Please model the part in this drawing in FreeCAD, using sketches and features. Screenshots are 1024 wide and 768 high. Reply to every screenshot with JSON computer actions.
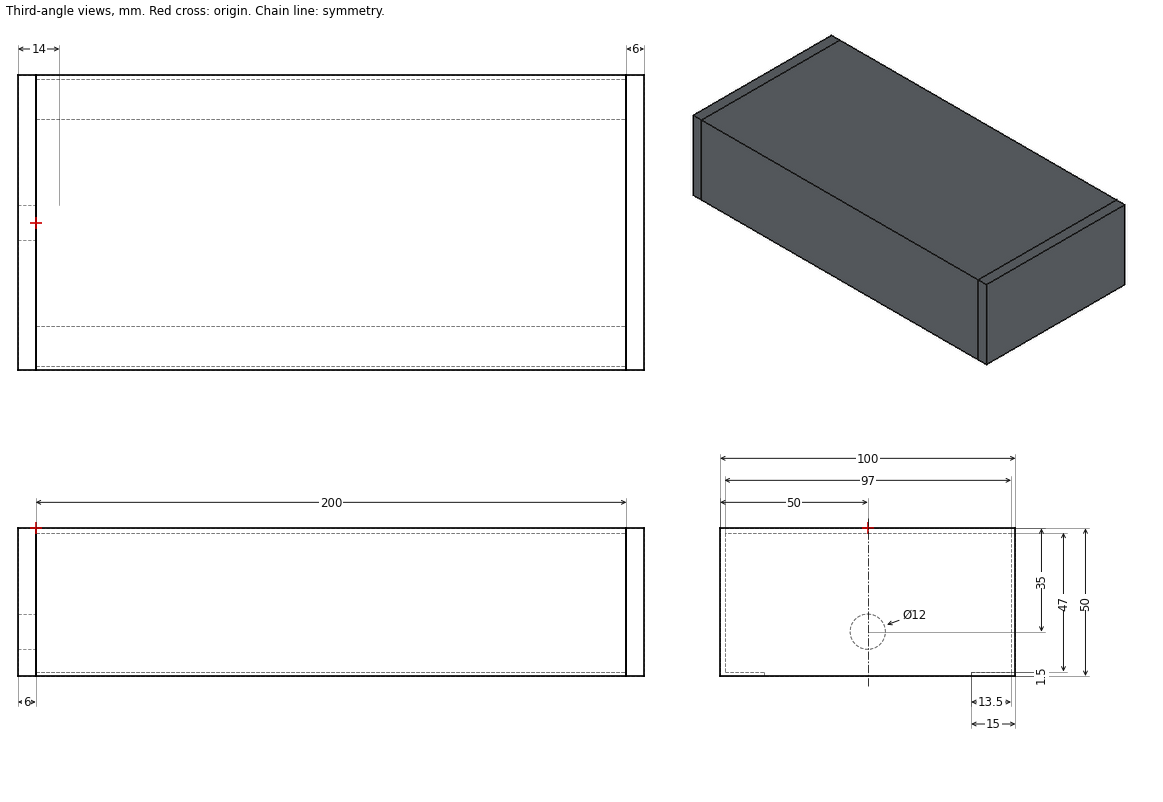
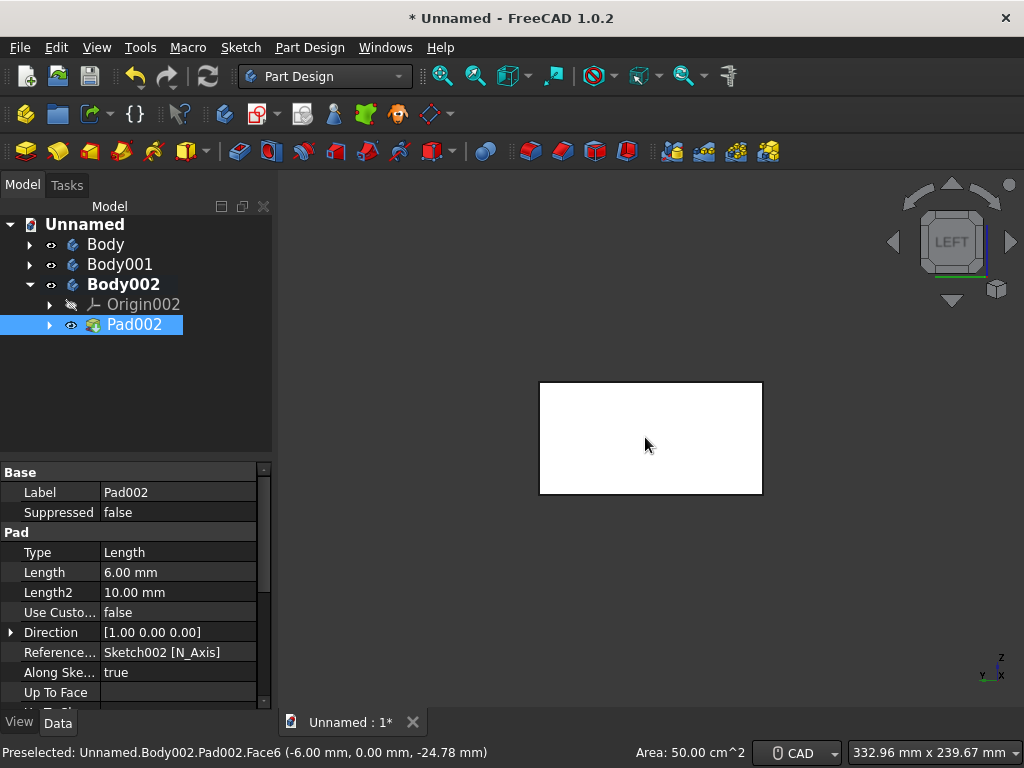
{"action": "left_click", "coordinate": [258, 114]}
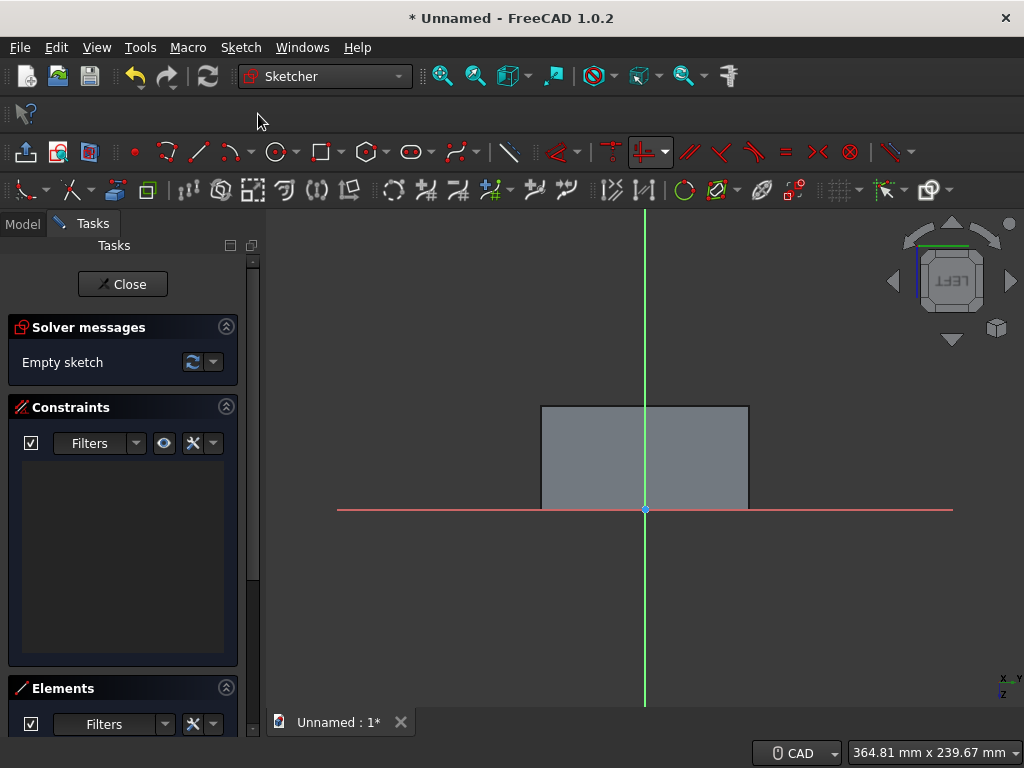
{"action": "scroll", "coordinate": [650, 436], "scroll_direction": "up", "scroll_amount": 13}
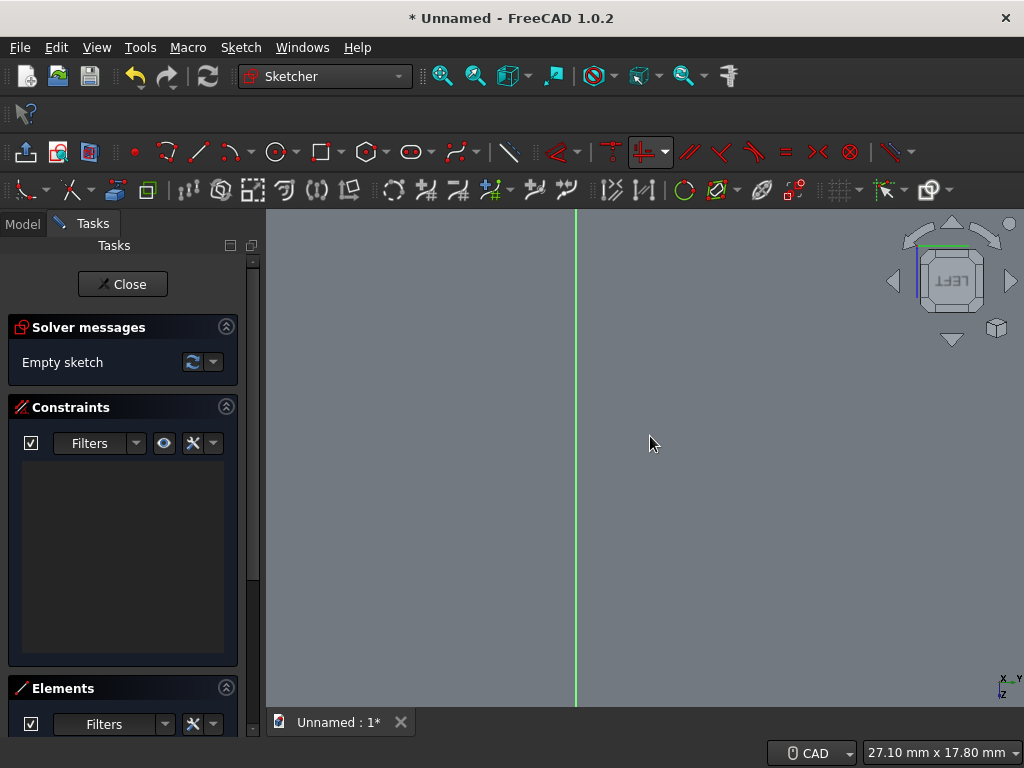
{"action": "left_click", "coordinate": [276, 152]}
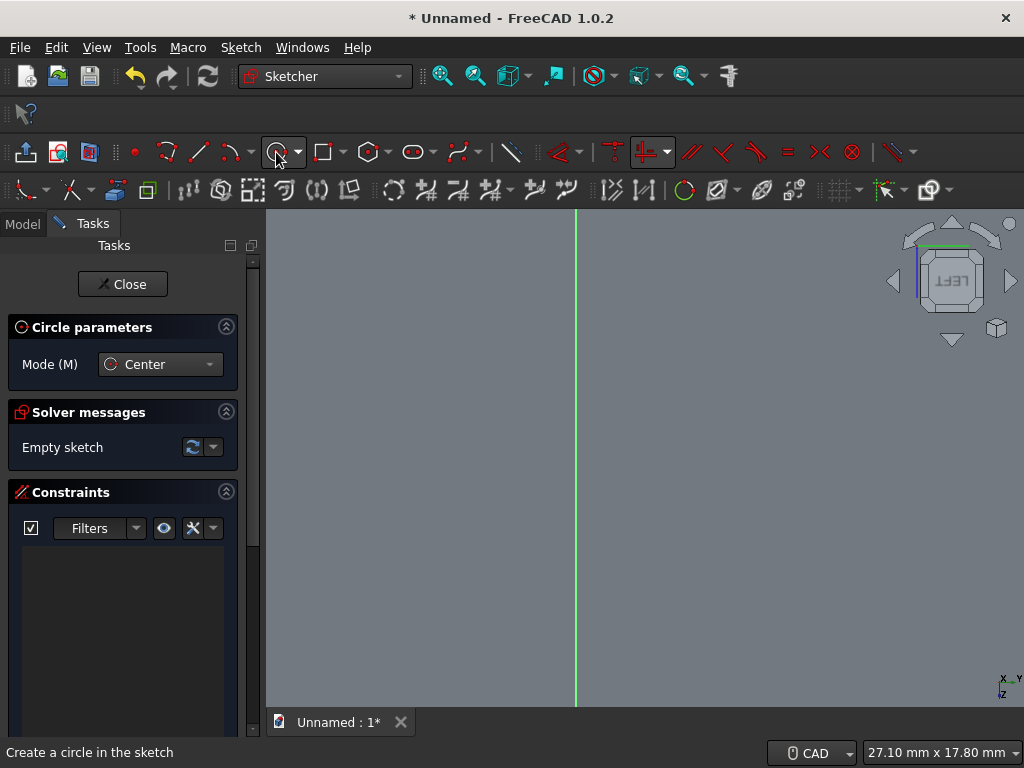
{"action": "left_click", "coordinate": [576, 447]}
{"action": "mouse_move", "coordinate": [695, 328]}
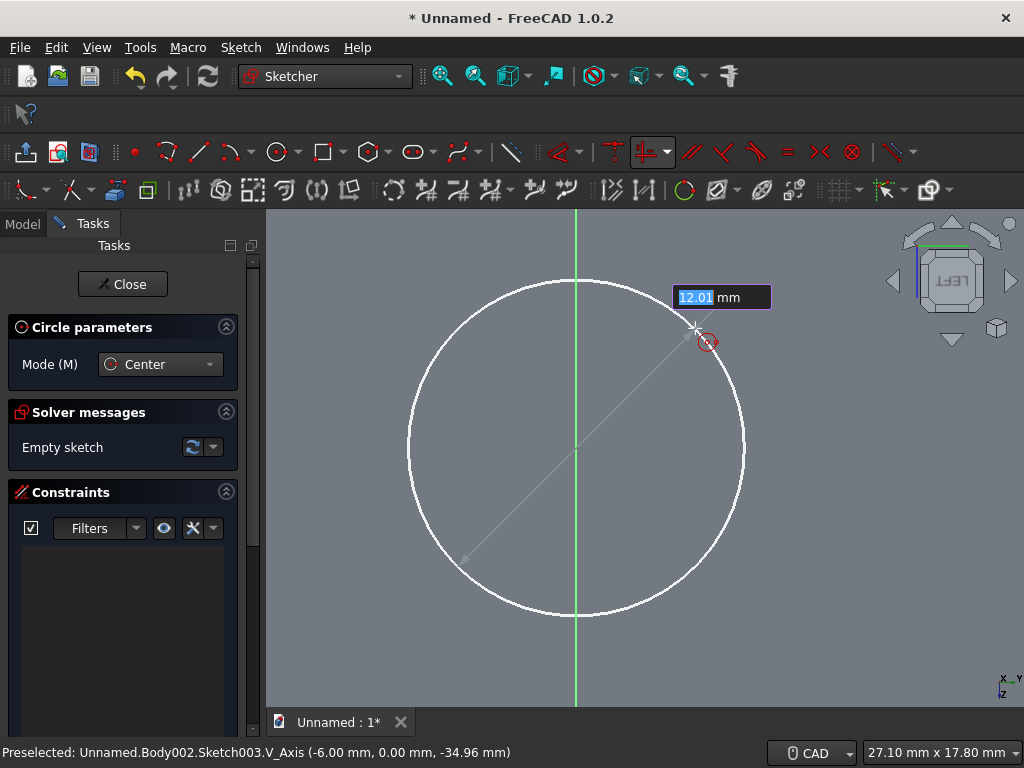
{"action": "type", "text": "12"}
{"action": "key", "text": "Return"}
{"action": "key", "text": "Escape"}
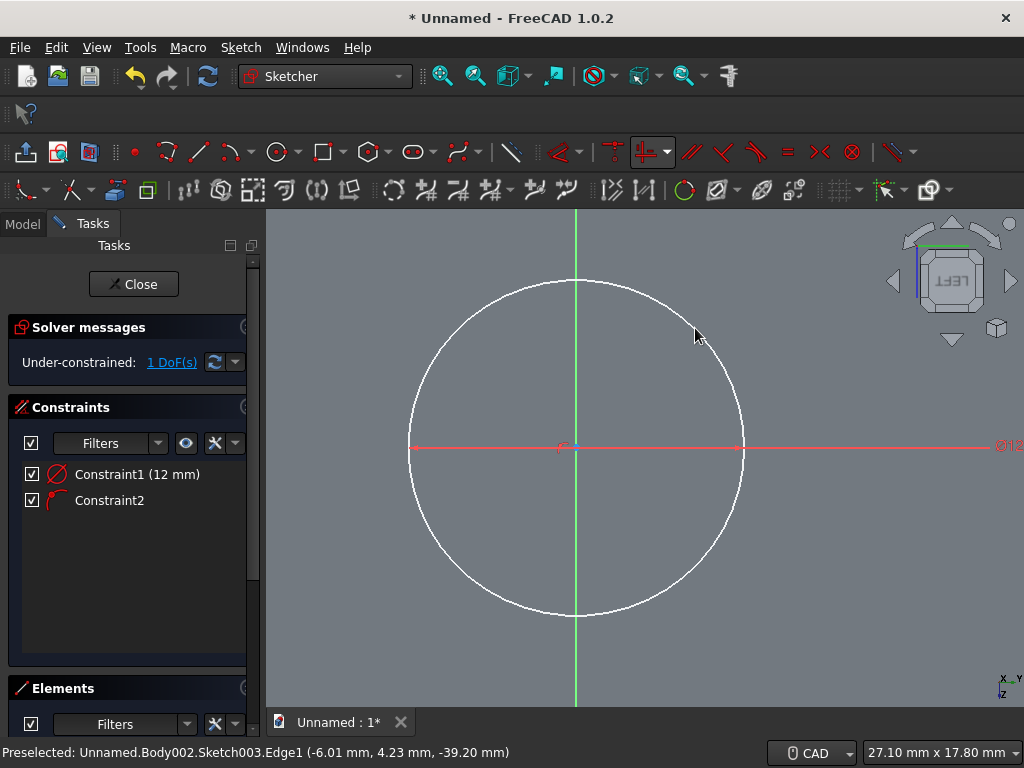
{"action": "left_click", "coordinate": [558, 152]}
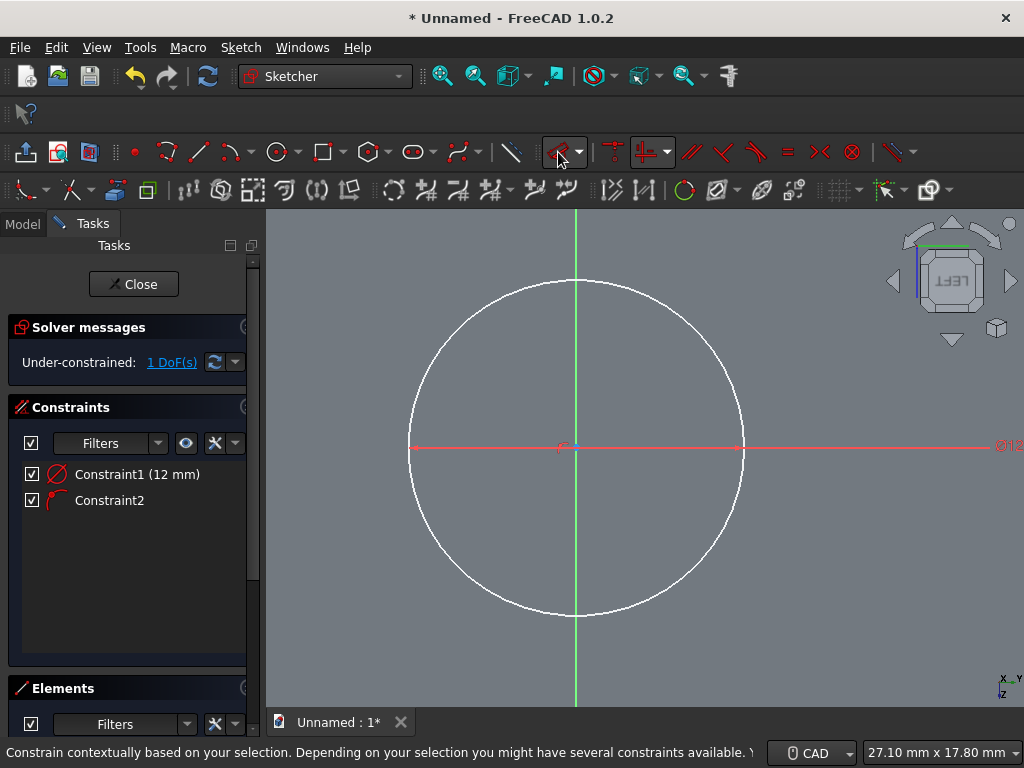
{"action": "left_click", "coordinate": [576, 448]}
{"action": "left_click", "coordinate": [610, 563]}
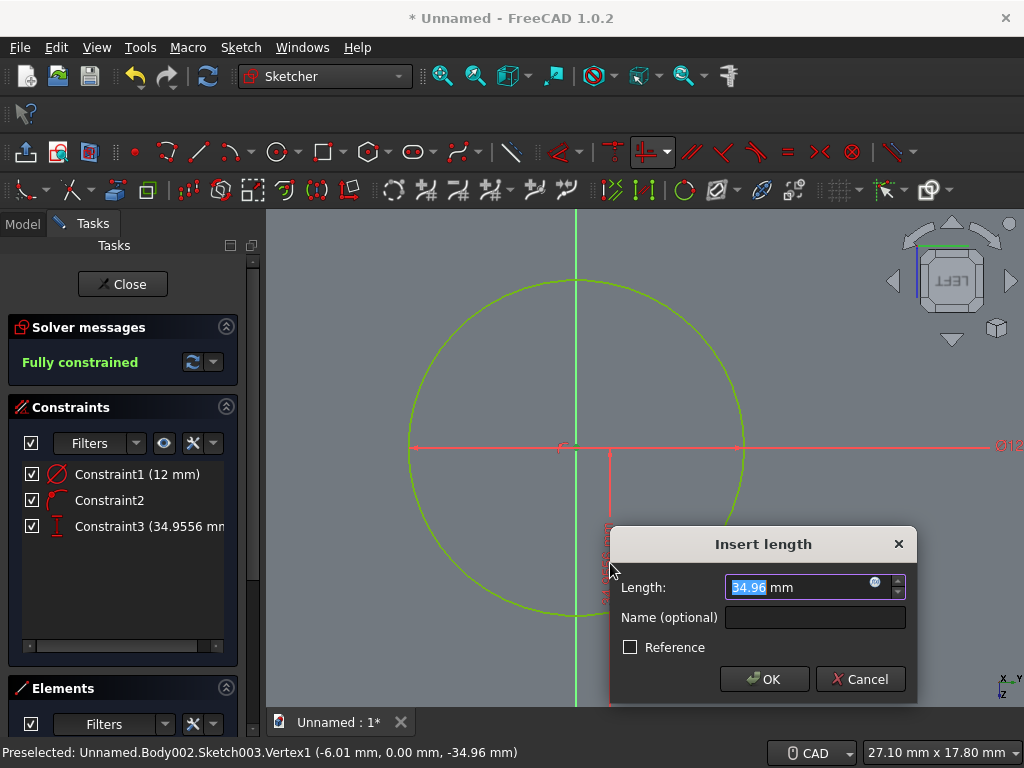
{"action": "type", "text": "35"}
{"action": "key", "text": "Return"}
{"action": "key", "text": "Escape"}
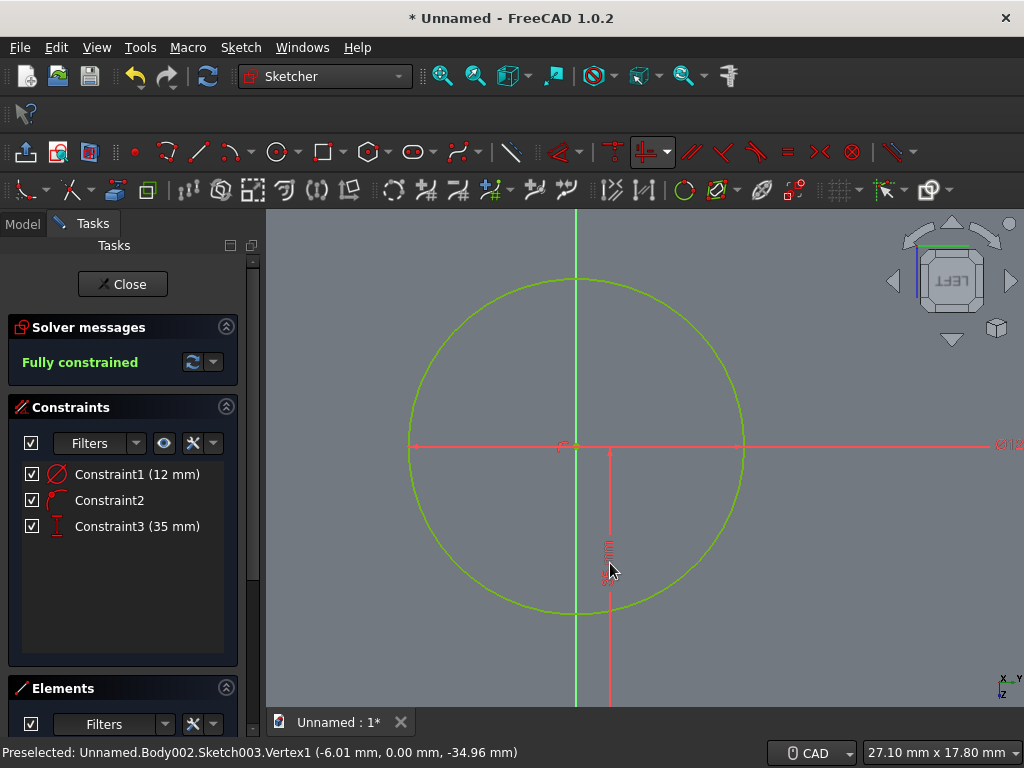
{"action": "left_click", "coordinate": [123, 284]}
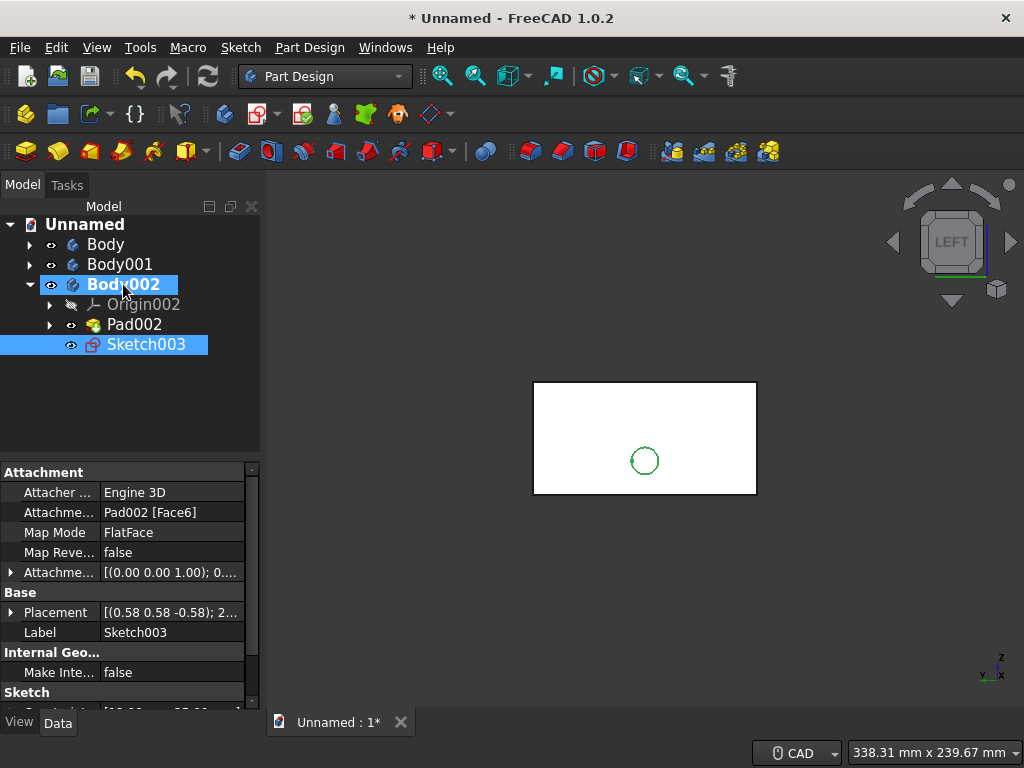
{"action": "left_click", "coordinate": [240, 152]}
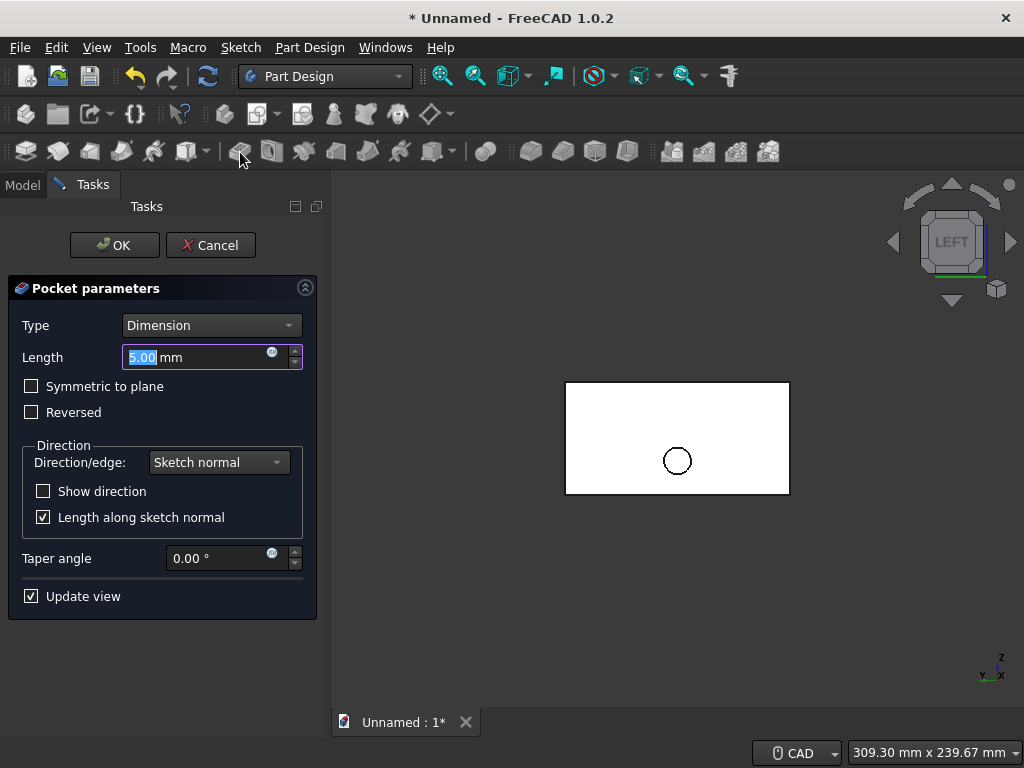
{"action": "type", "text": "14"}
{"action": "key", "text": "Tab"}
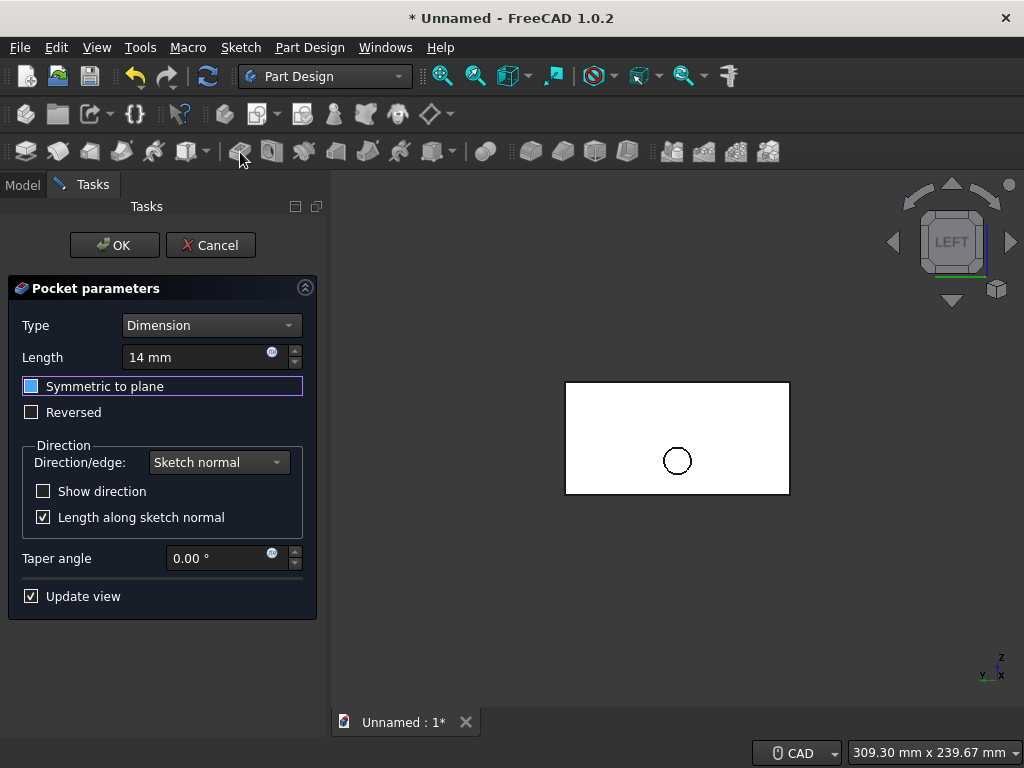
{"action": "left_click", "coordinate": [115, 245]}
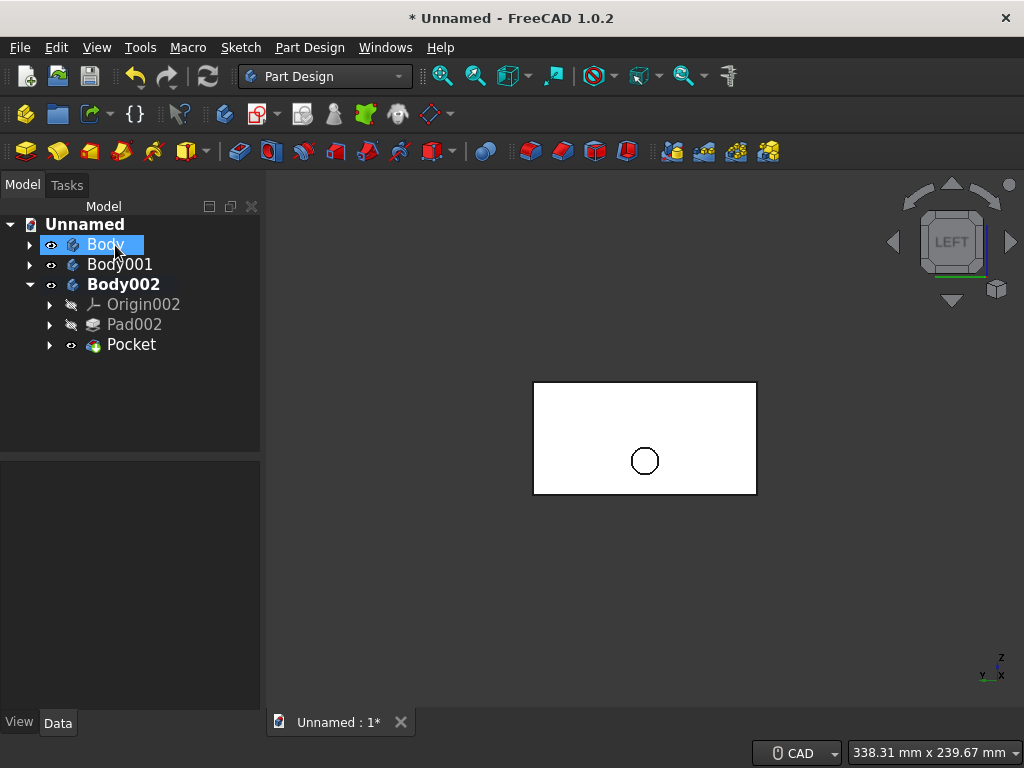
{"action": "key", "text": "0"}